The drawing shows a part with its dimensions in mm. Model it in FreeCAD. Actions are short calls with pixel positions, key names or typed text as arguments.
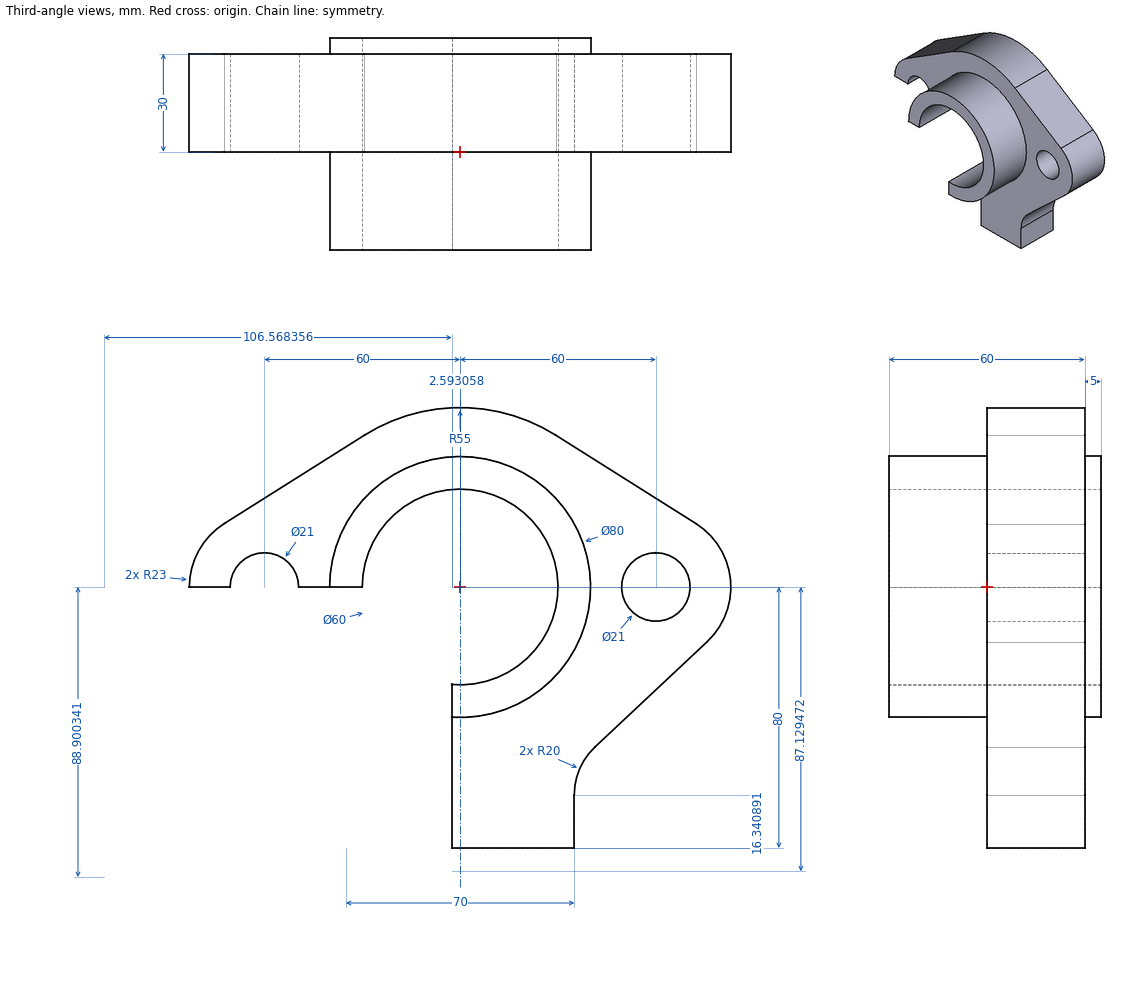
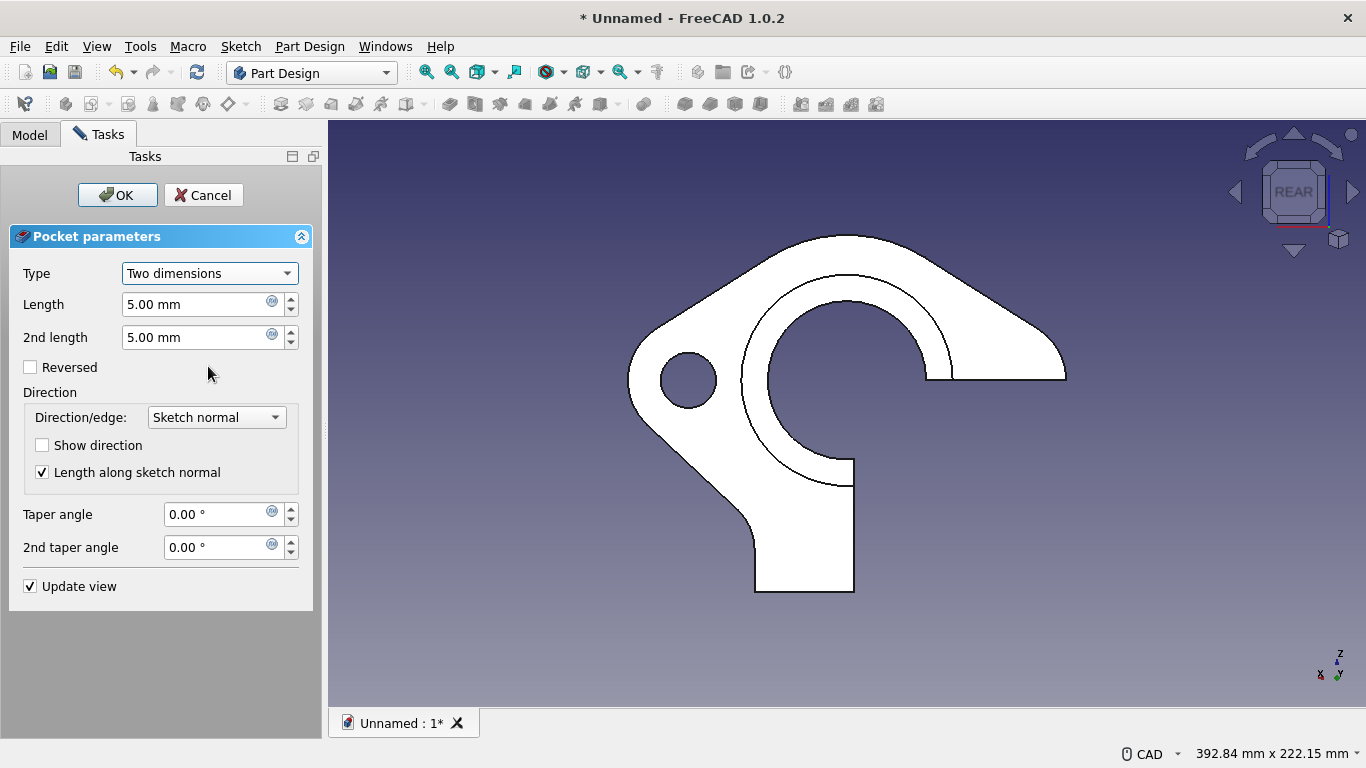
triple_click(204, 304)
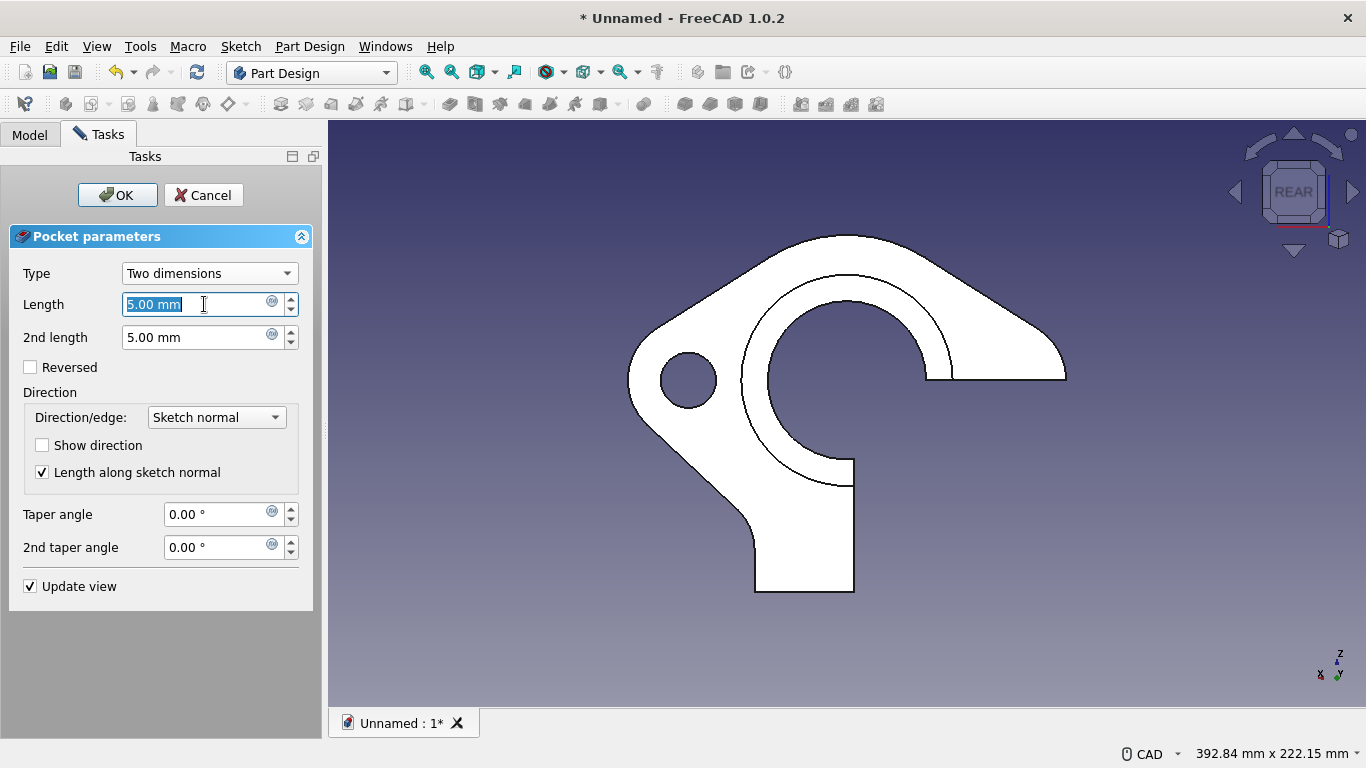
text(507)
key(Tab)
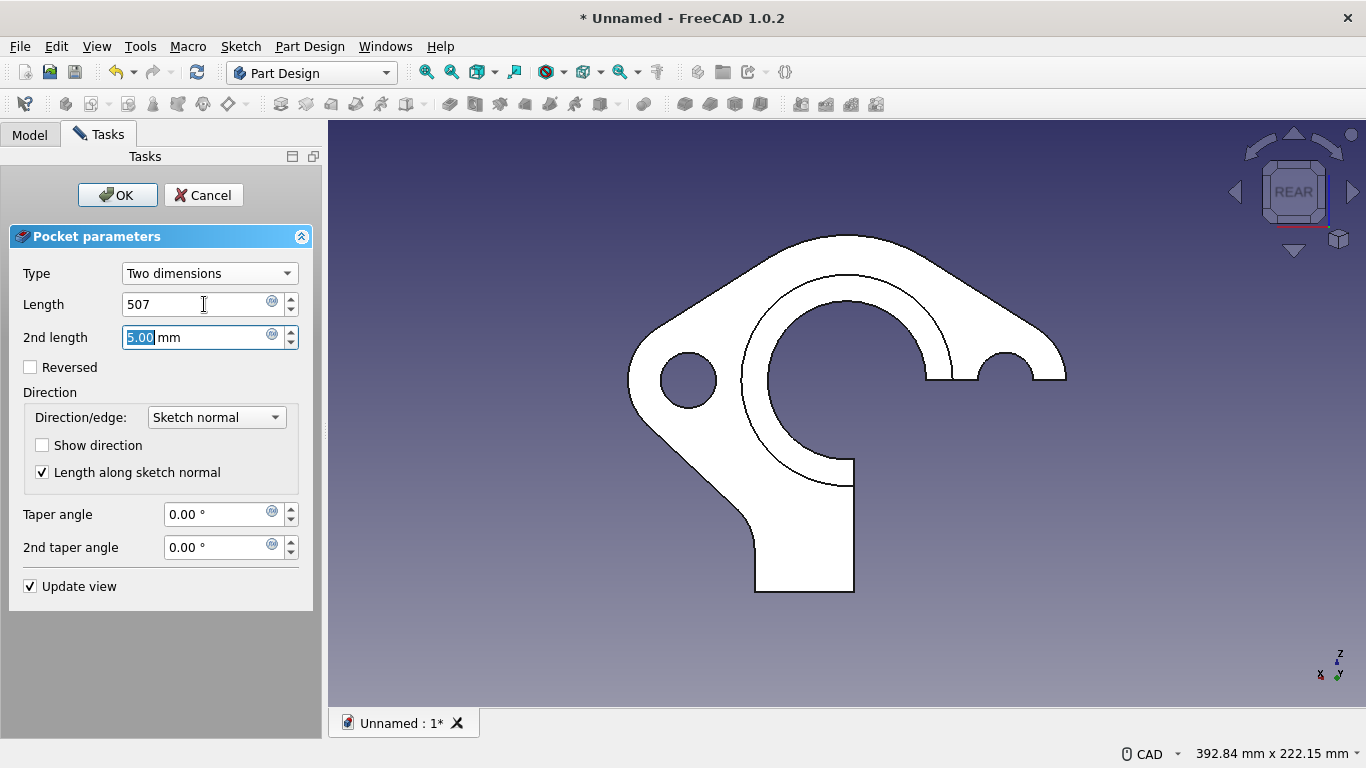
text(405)
key(Tab)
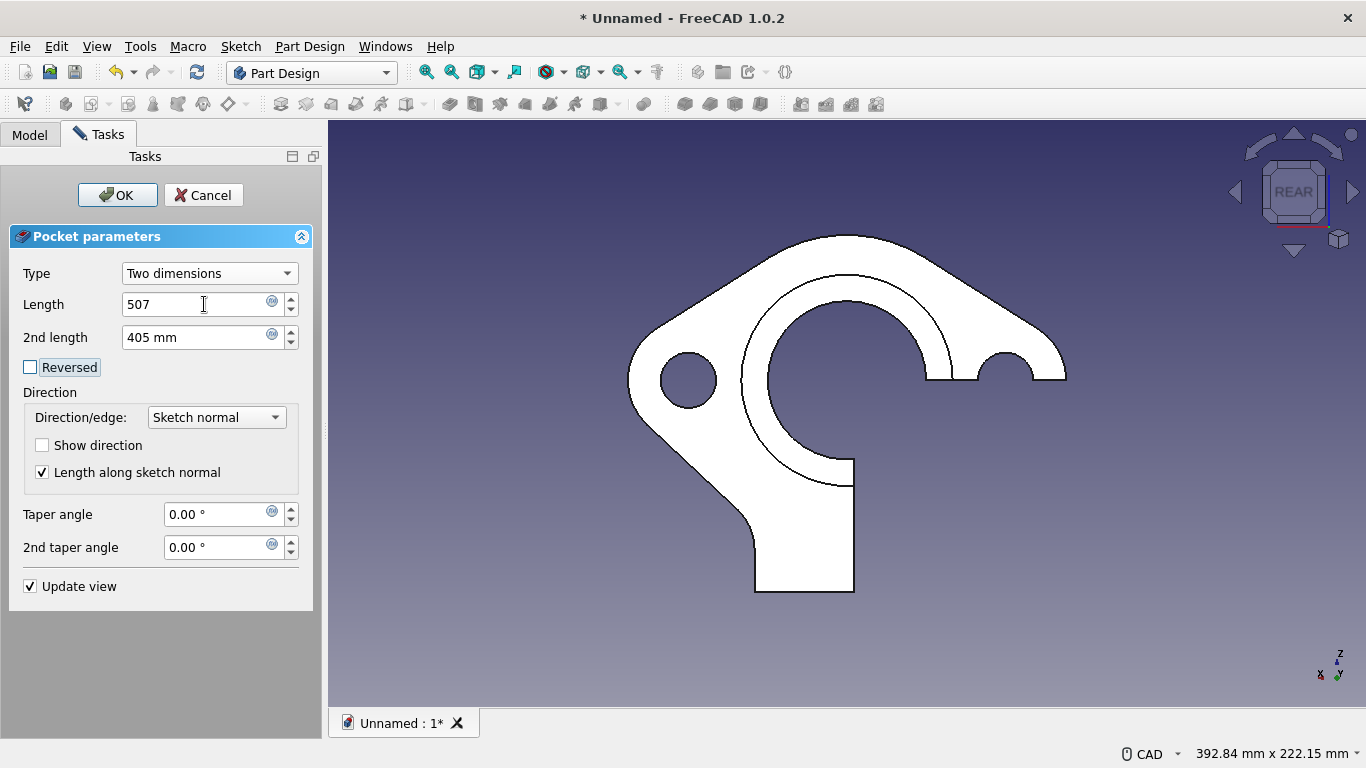
click(31, 367)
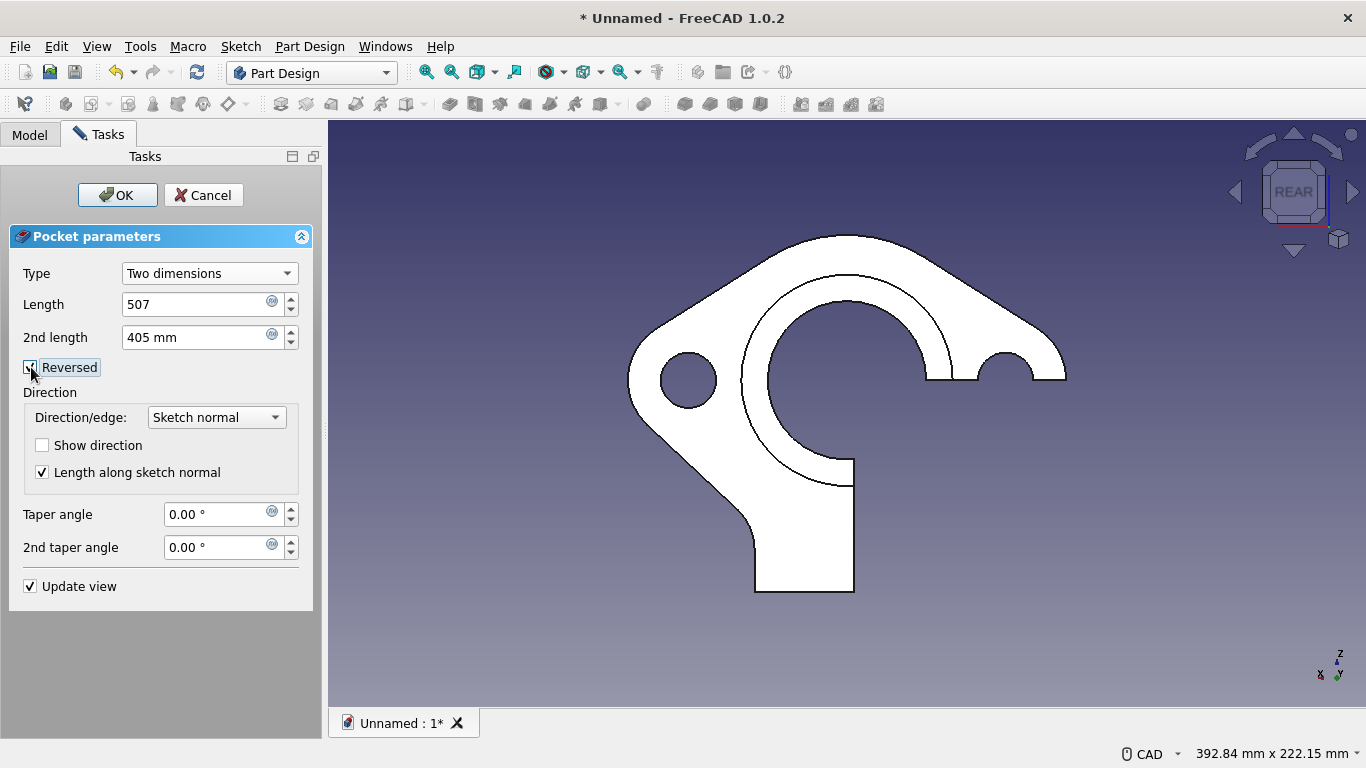
click(118, 195)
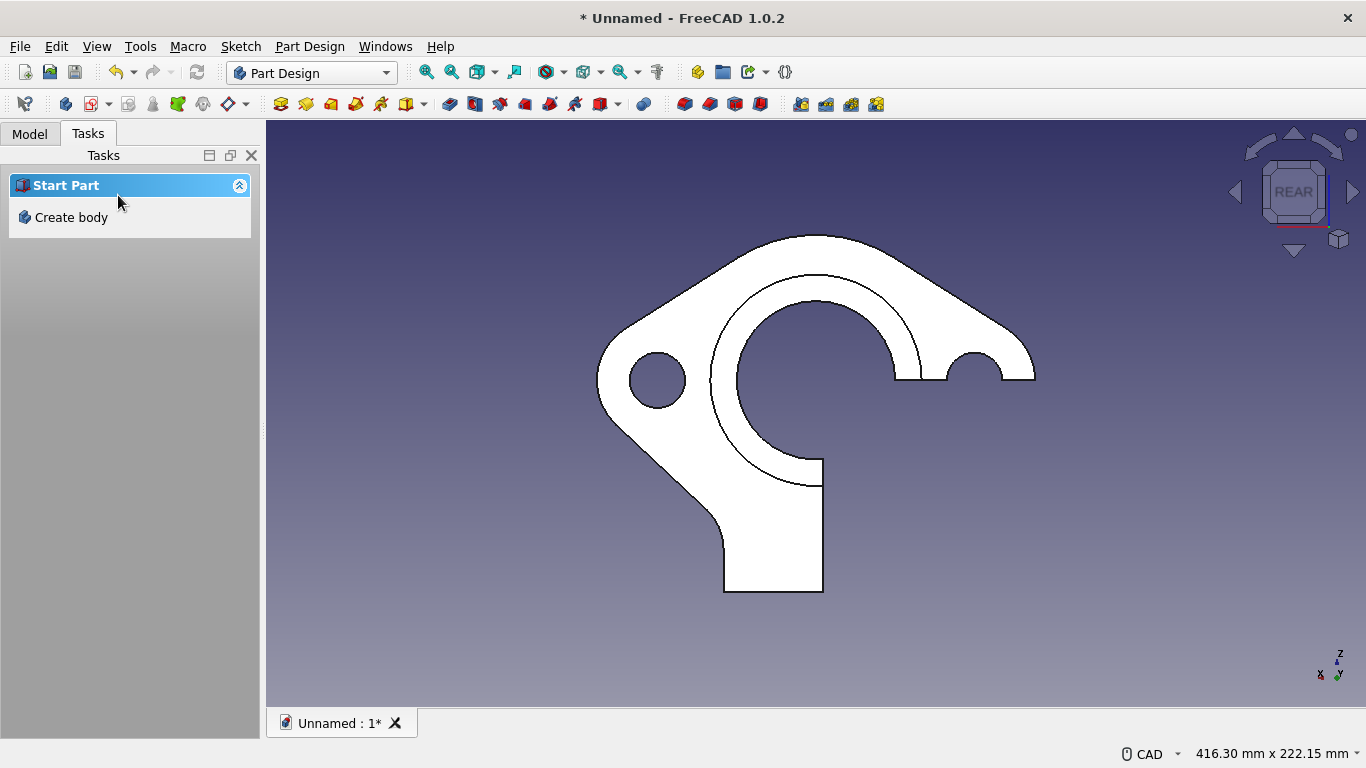
key(0)